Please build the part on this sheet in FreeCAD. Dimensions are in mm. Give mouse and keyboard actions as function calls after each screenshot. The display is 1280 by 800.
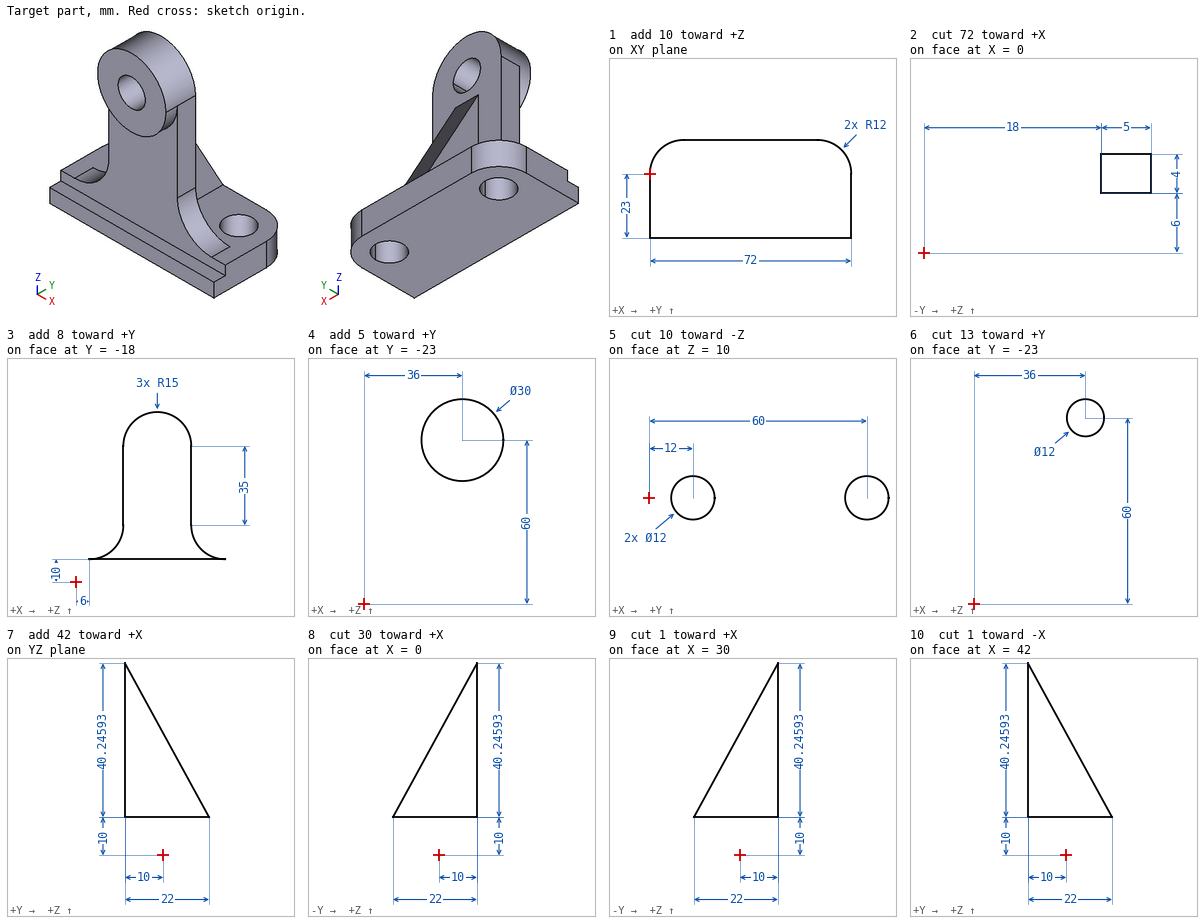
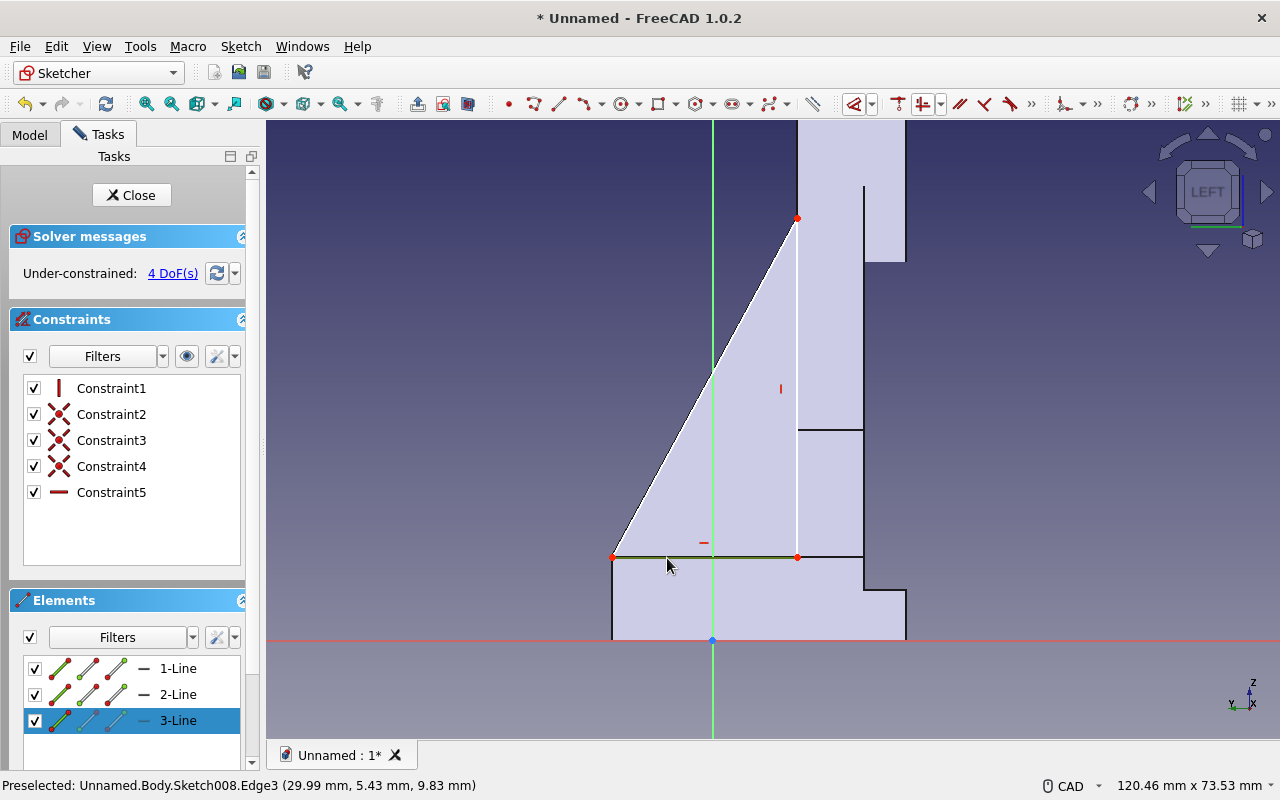
key(l)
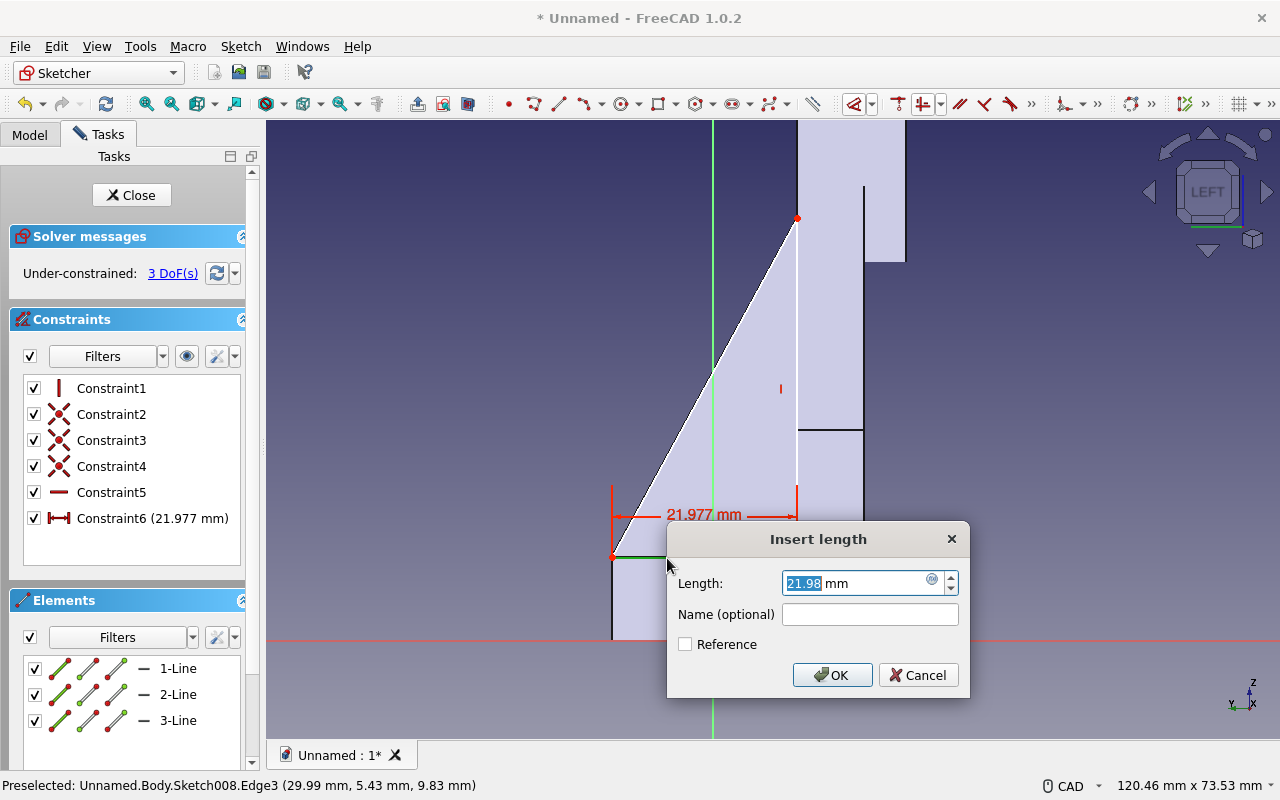
text(22)
key(Return)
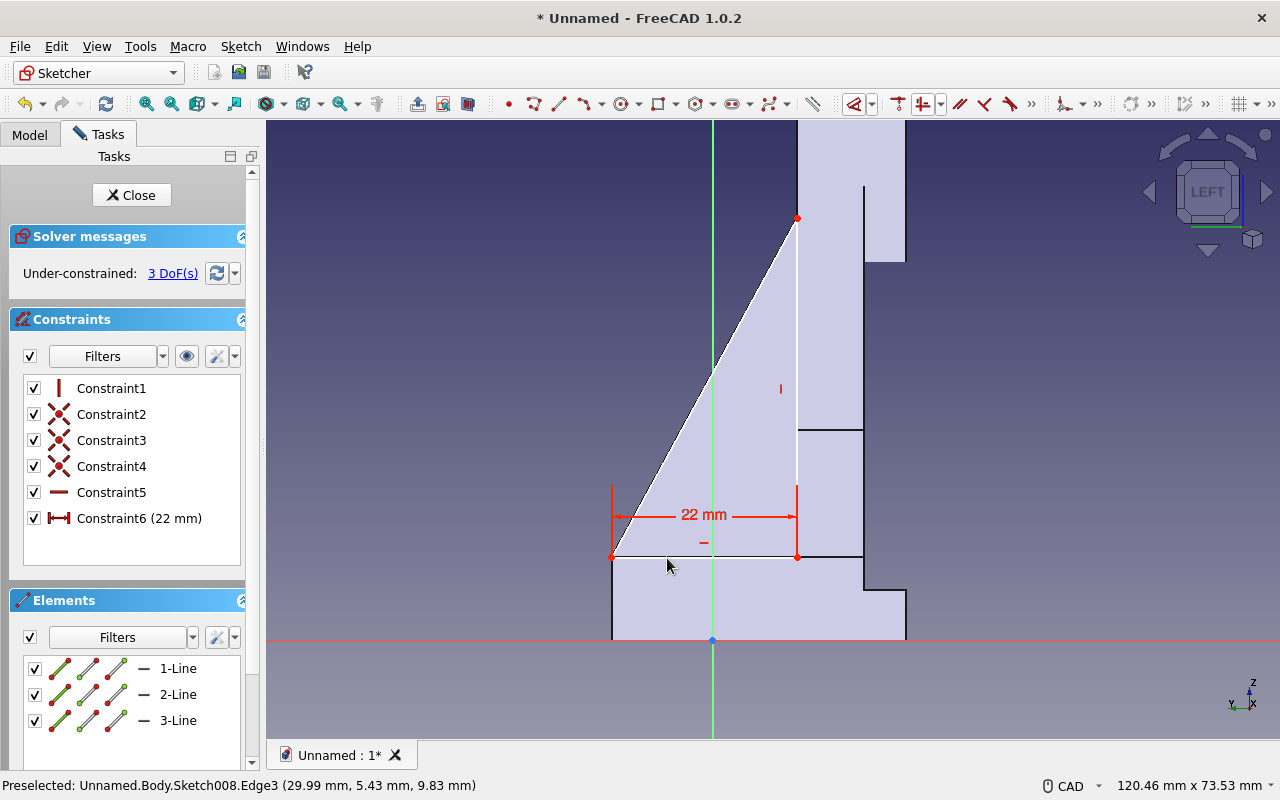
click(797, 558)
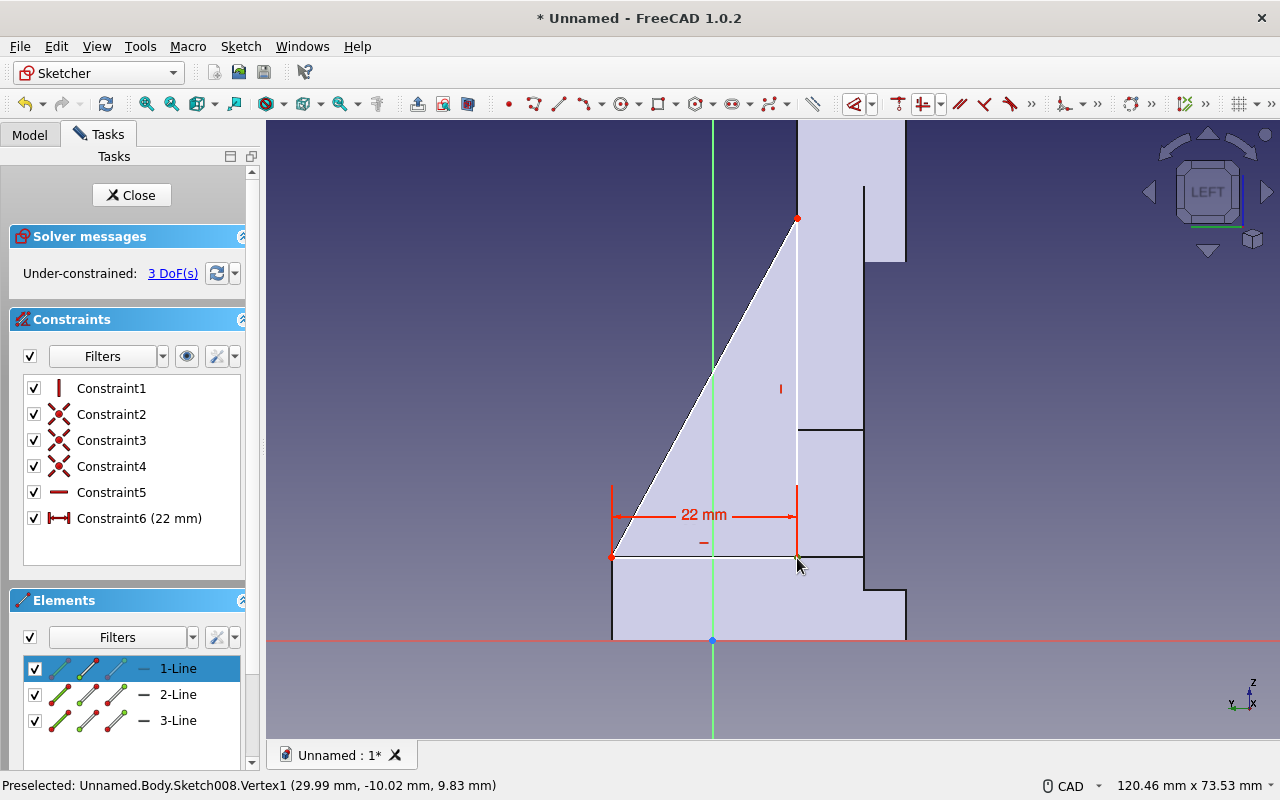
click(872, 104)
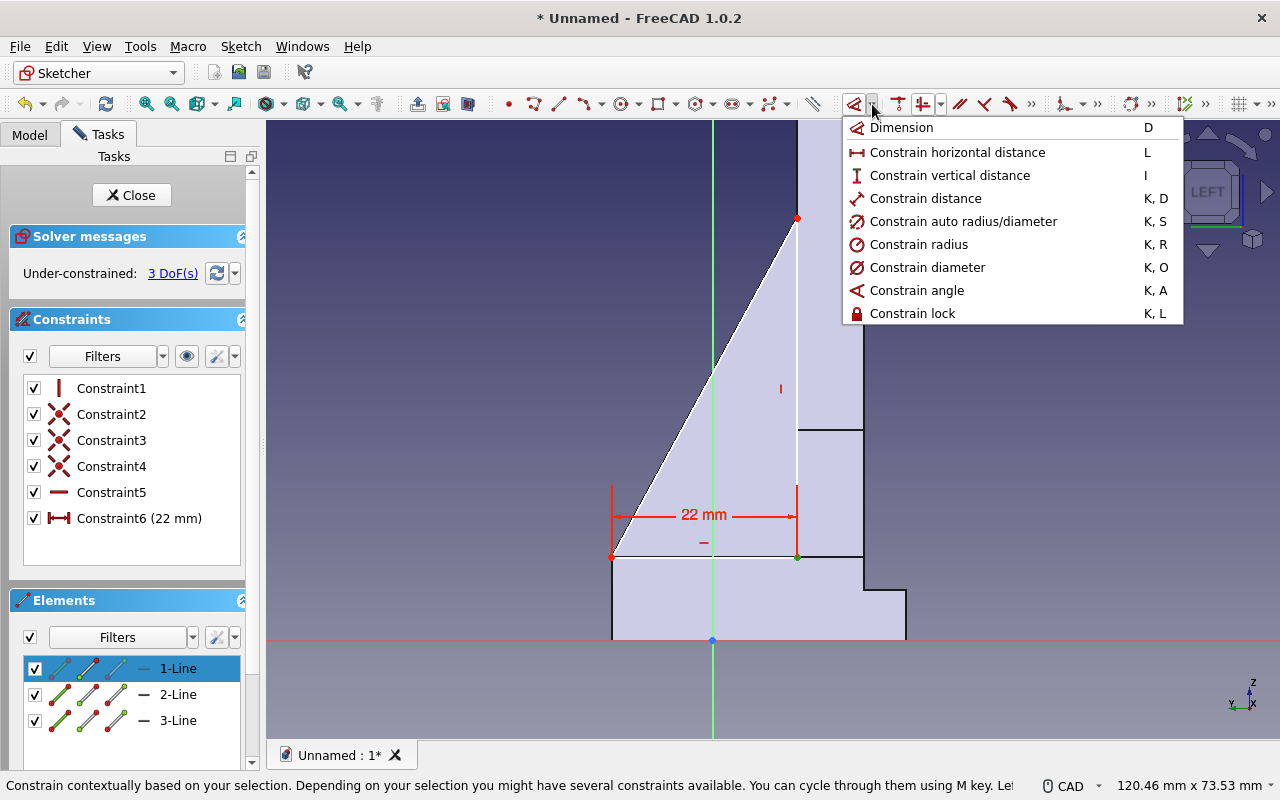
click(1013, 152)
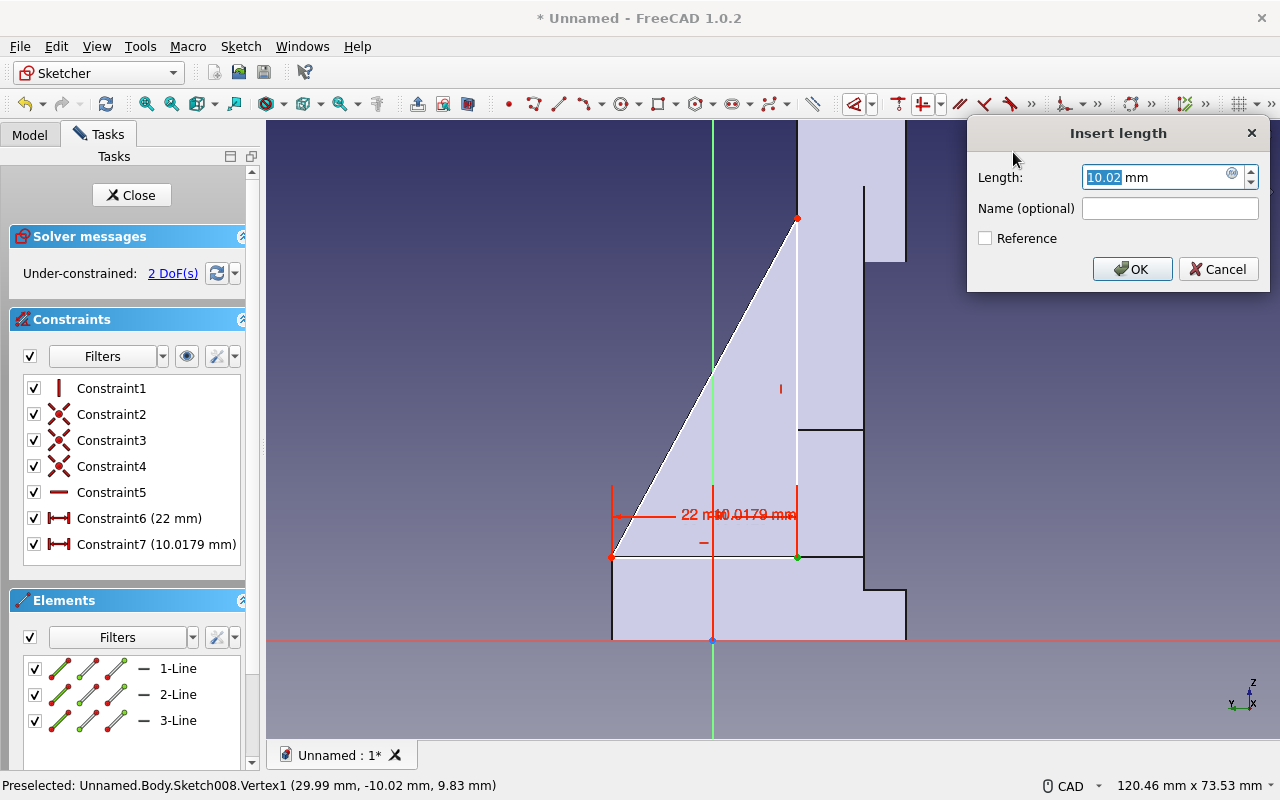
text(10)
key(Return)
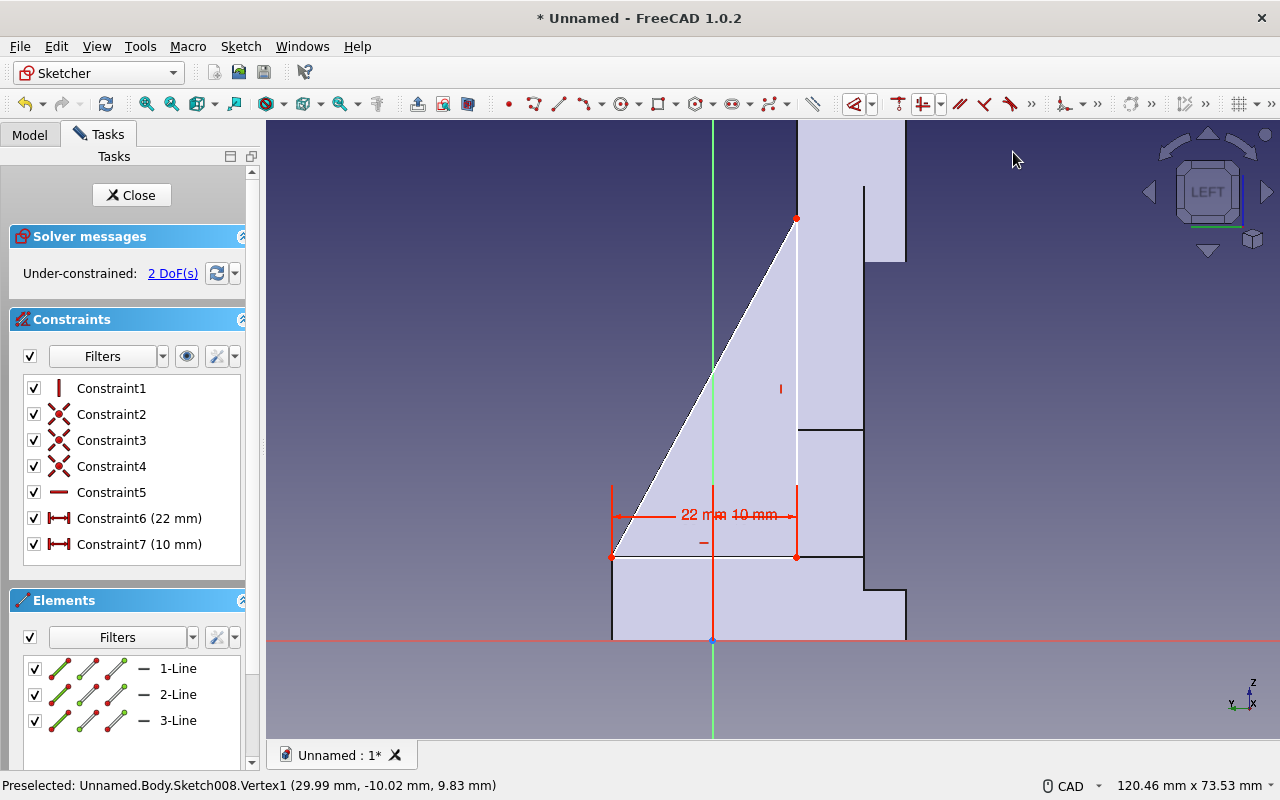
click(797, 558)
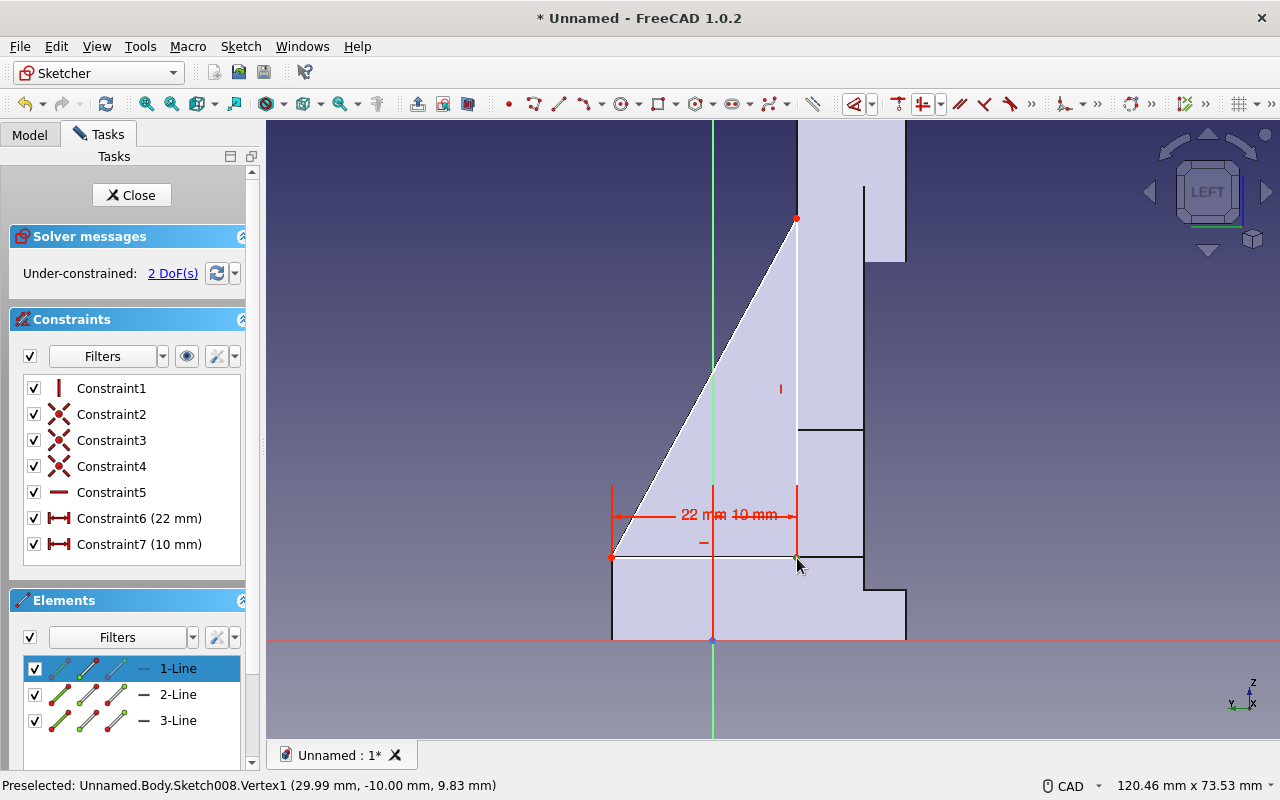
click(872, 104)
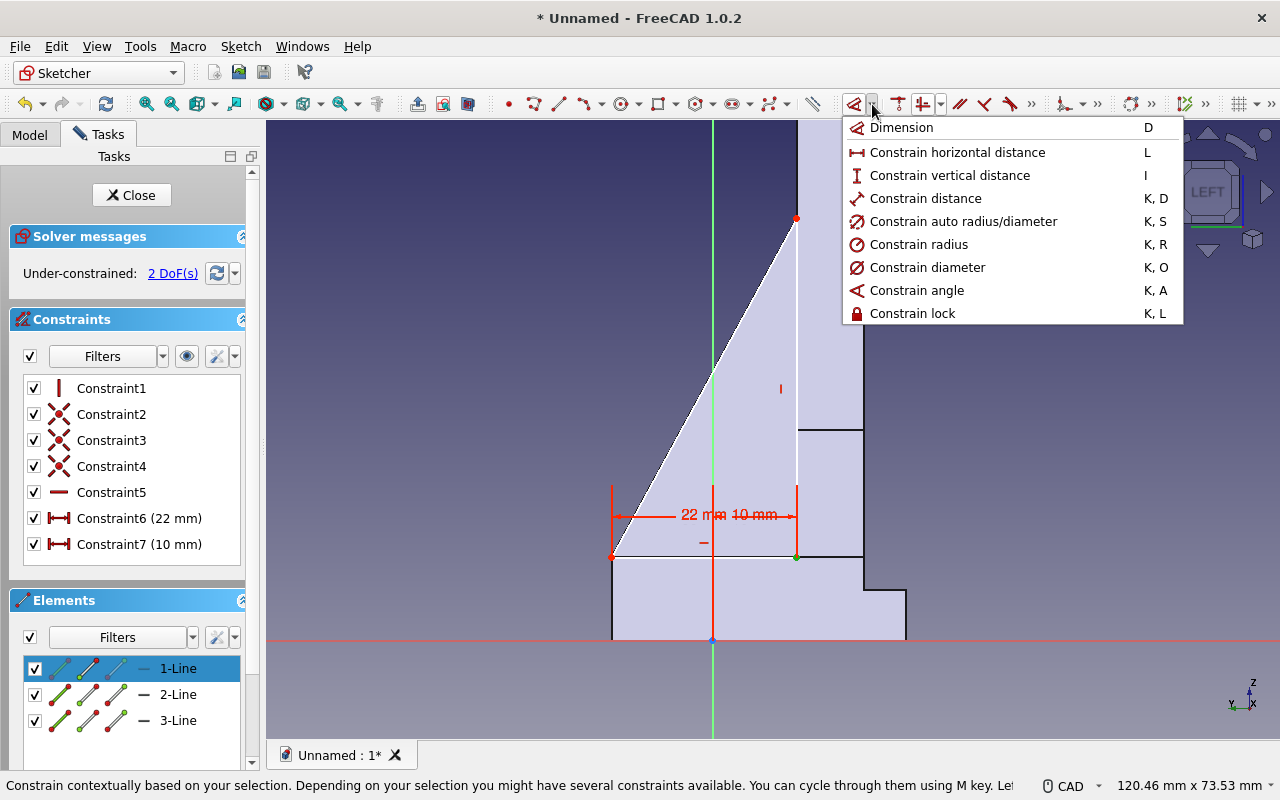
click(1013, 176)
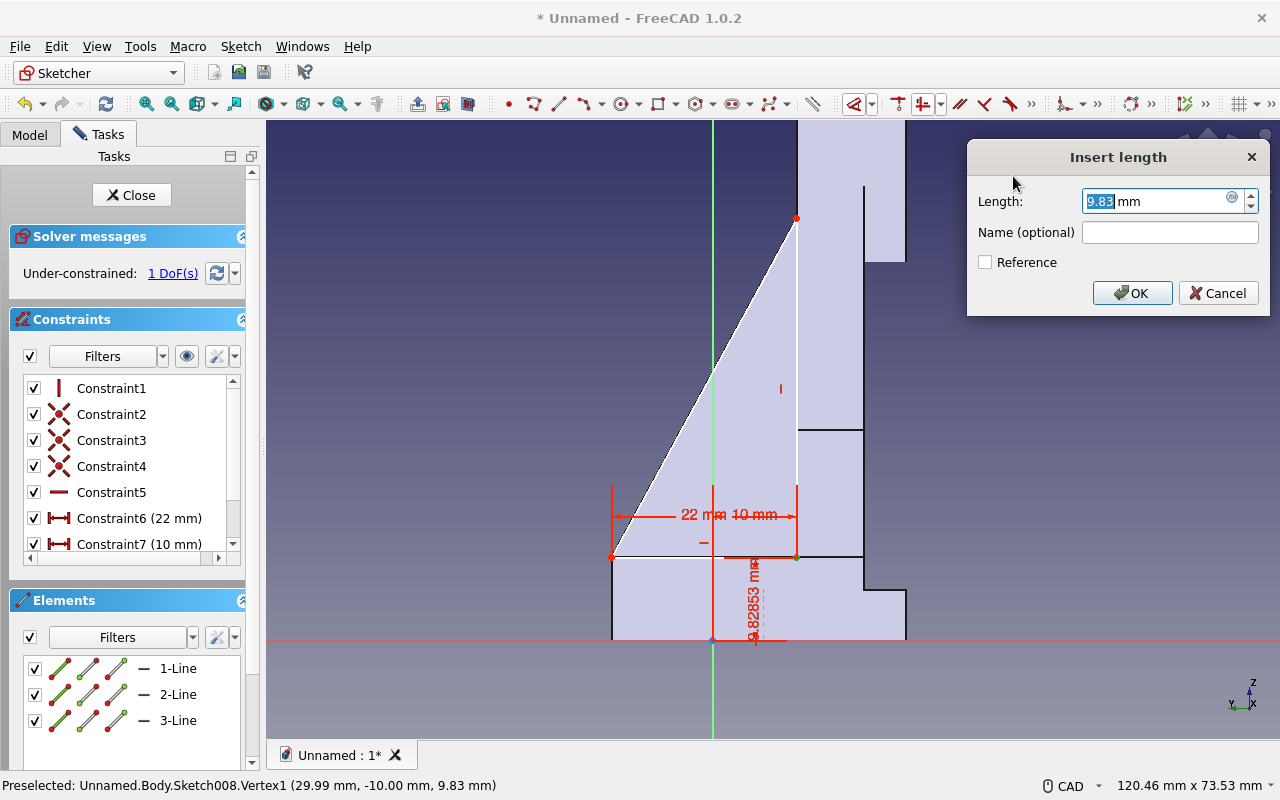
text(10)
key(Return)